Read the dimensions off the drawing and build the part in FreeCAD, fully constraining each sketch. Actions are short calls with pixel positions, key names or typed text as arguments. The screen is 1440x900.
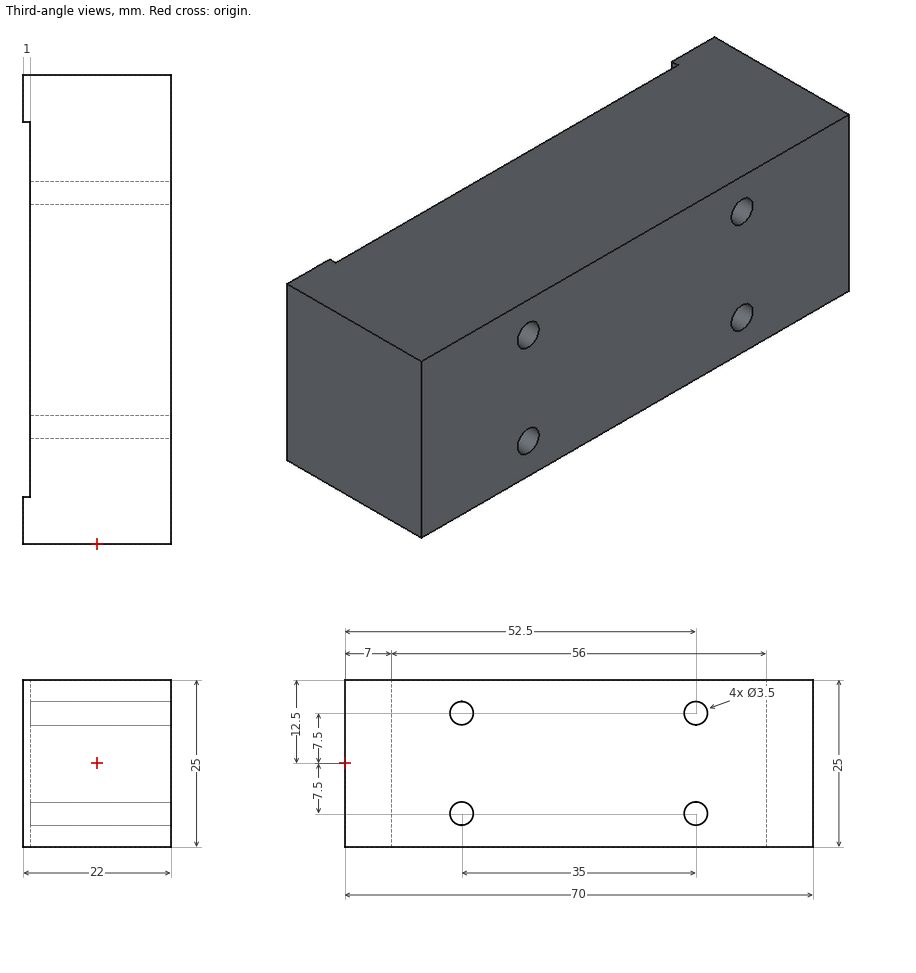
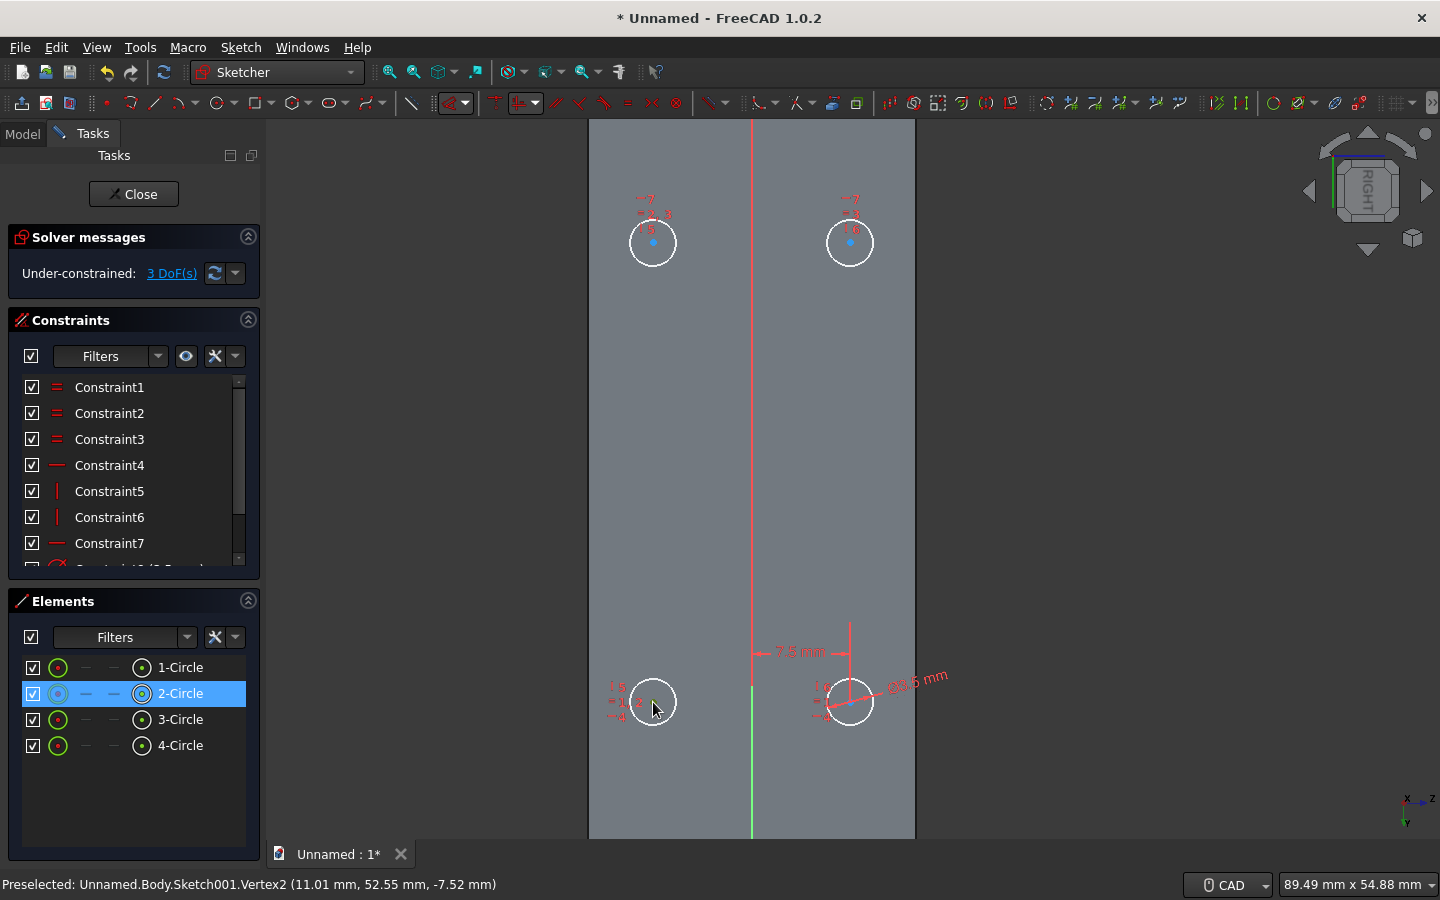
click(468, 104)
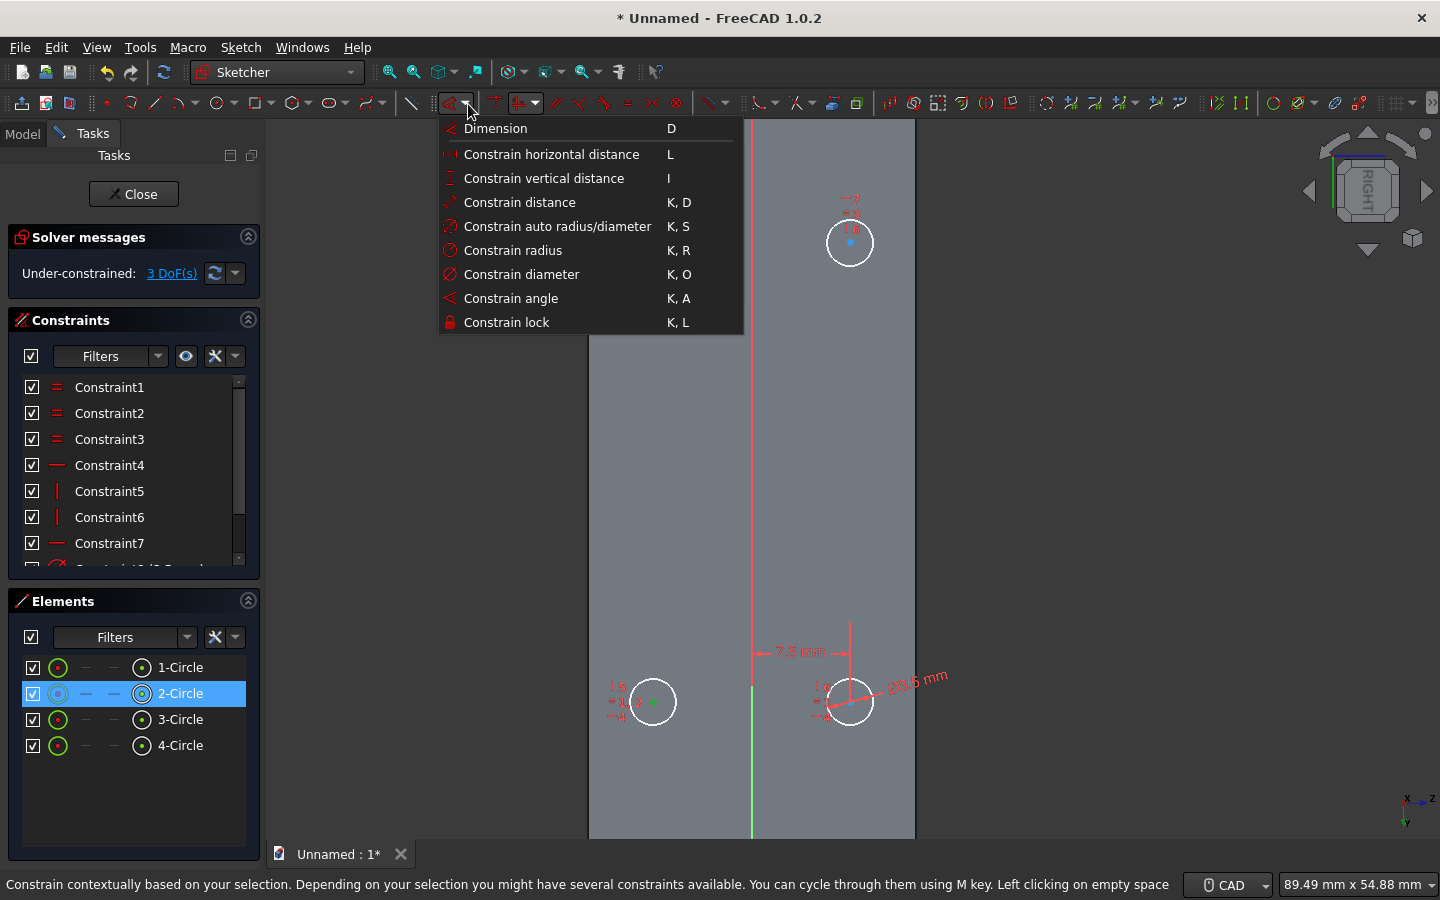
click(591, 154)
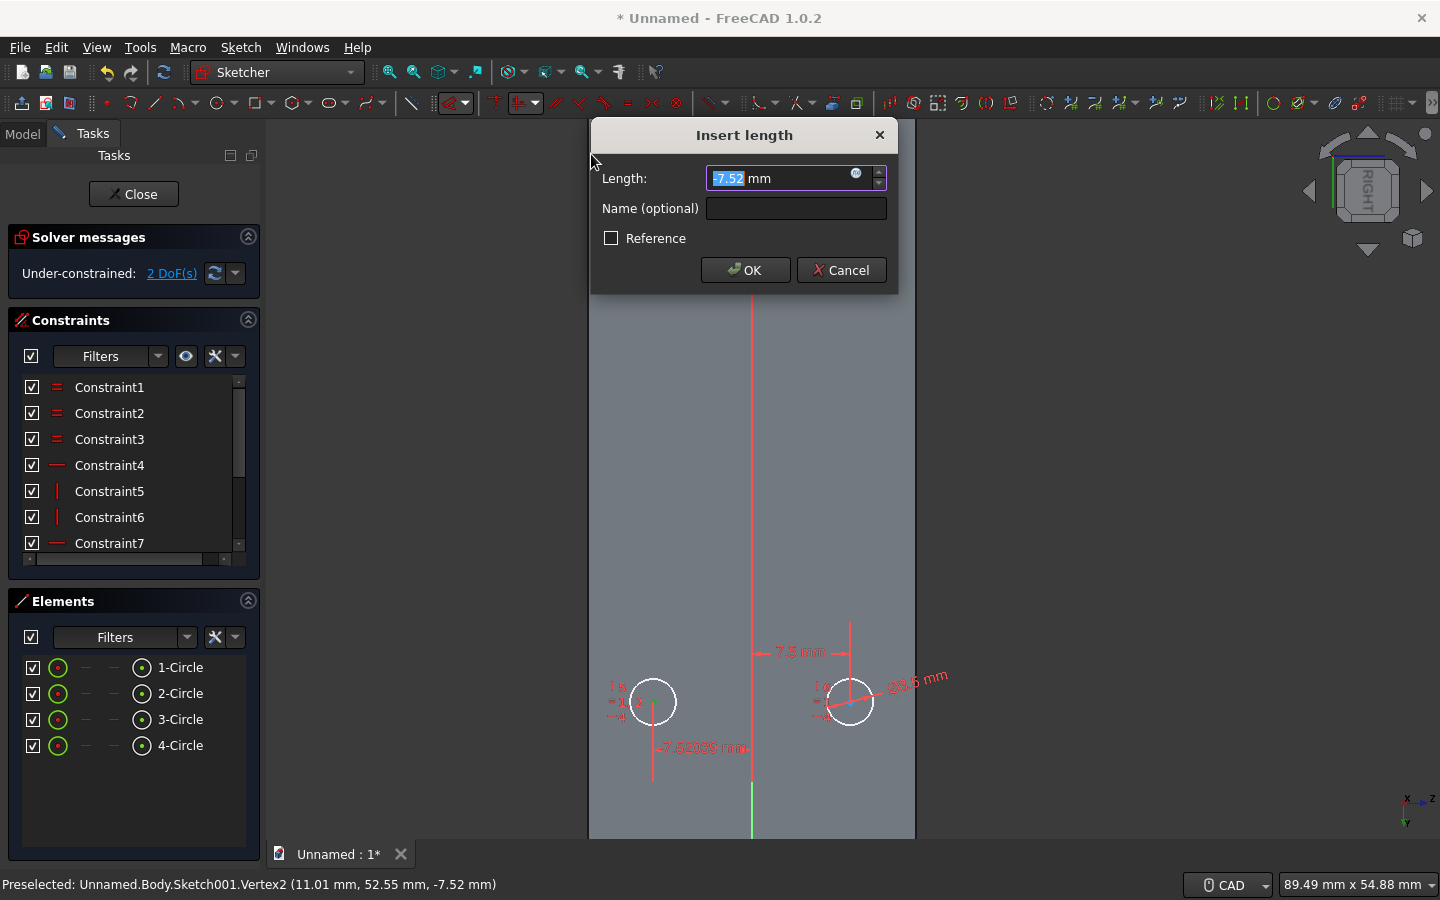
text(-7.5)
key(Return)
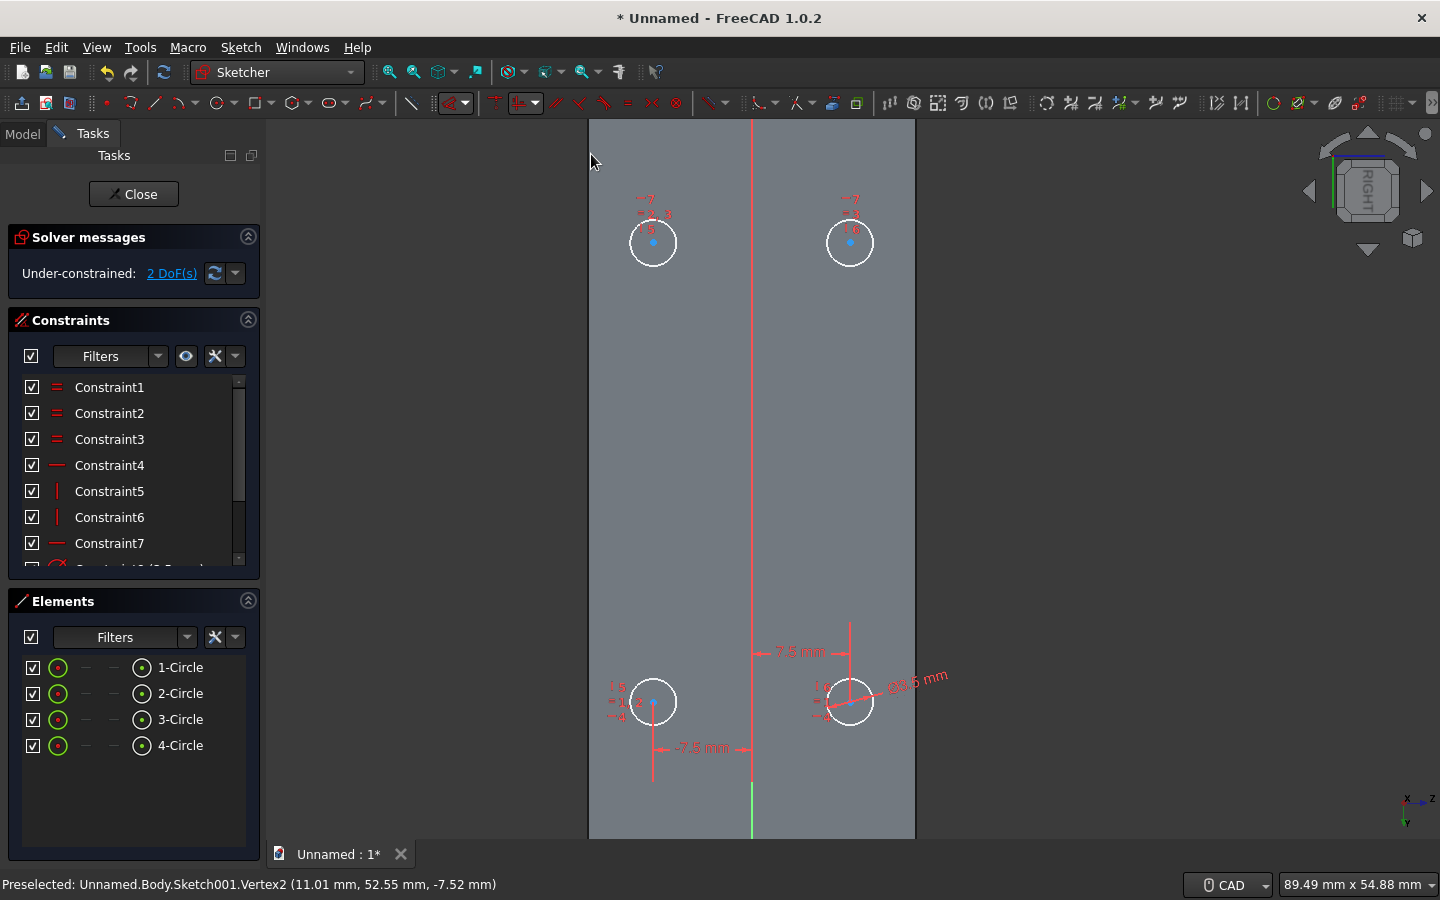
click(653, 702)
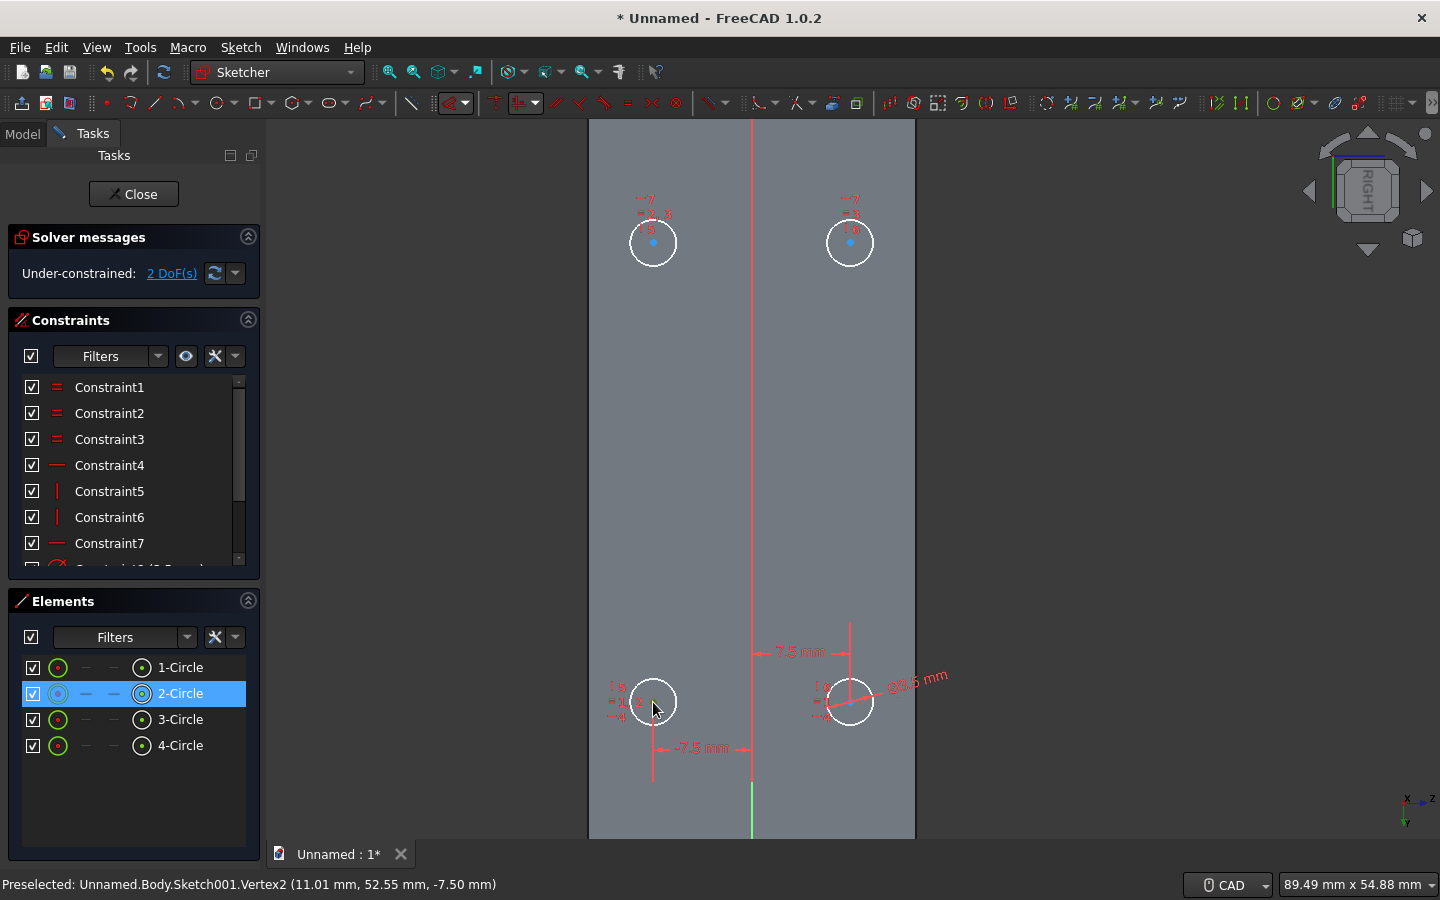
click(653, 243)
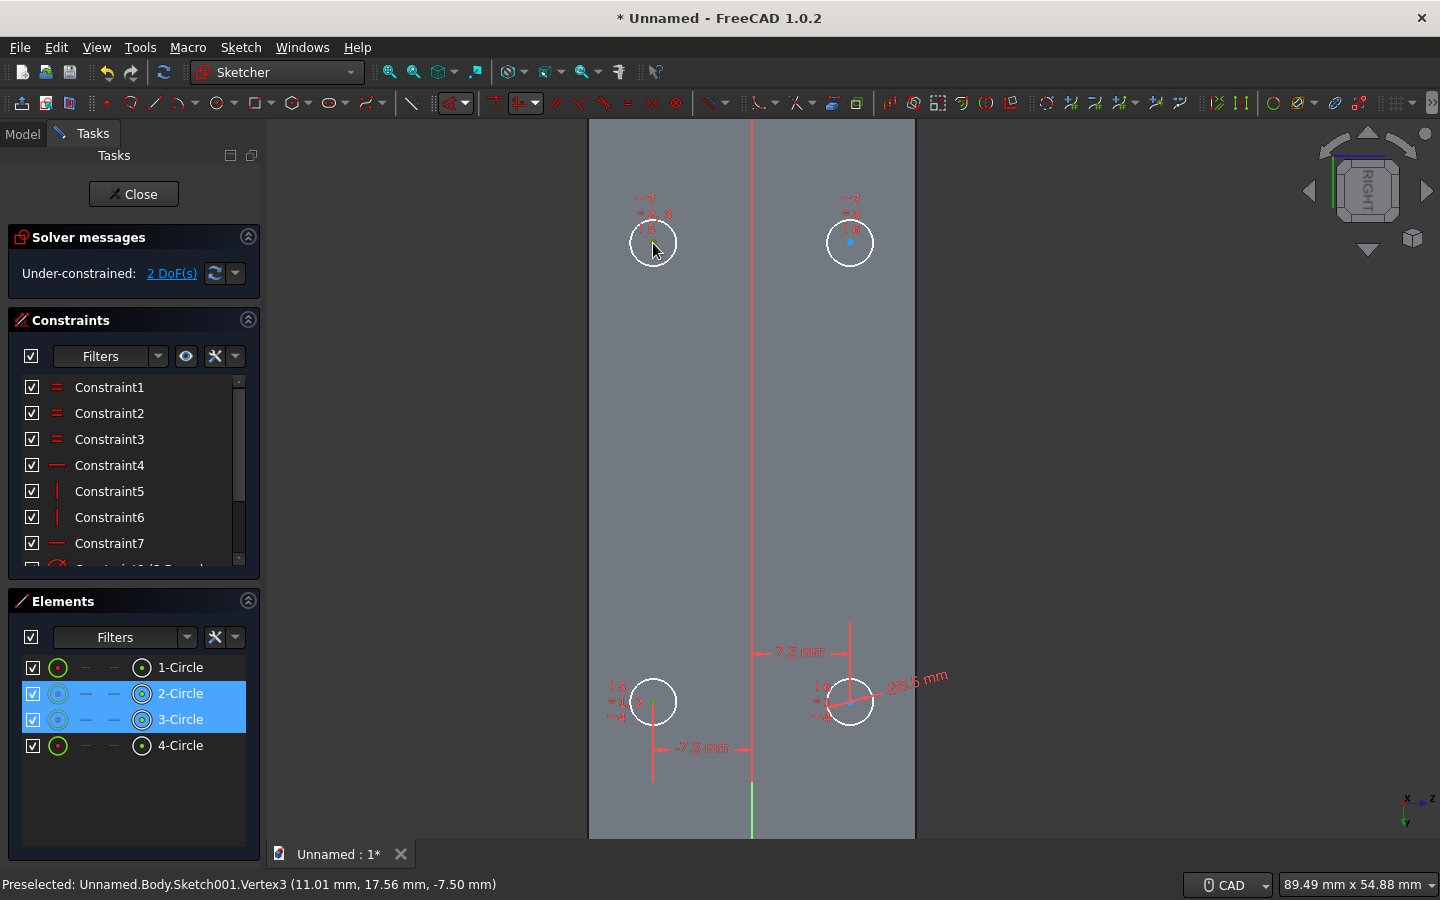
click(468, 104)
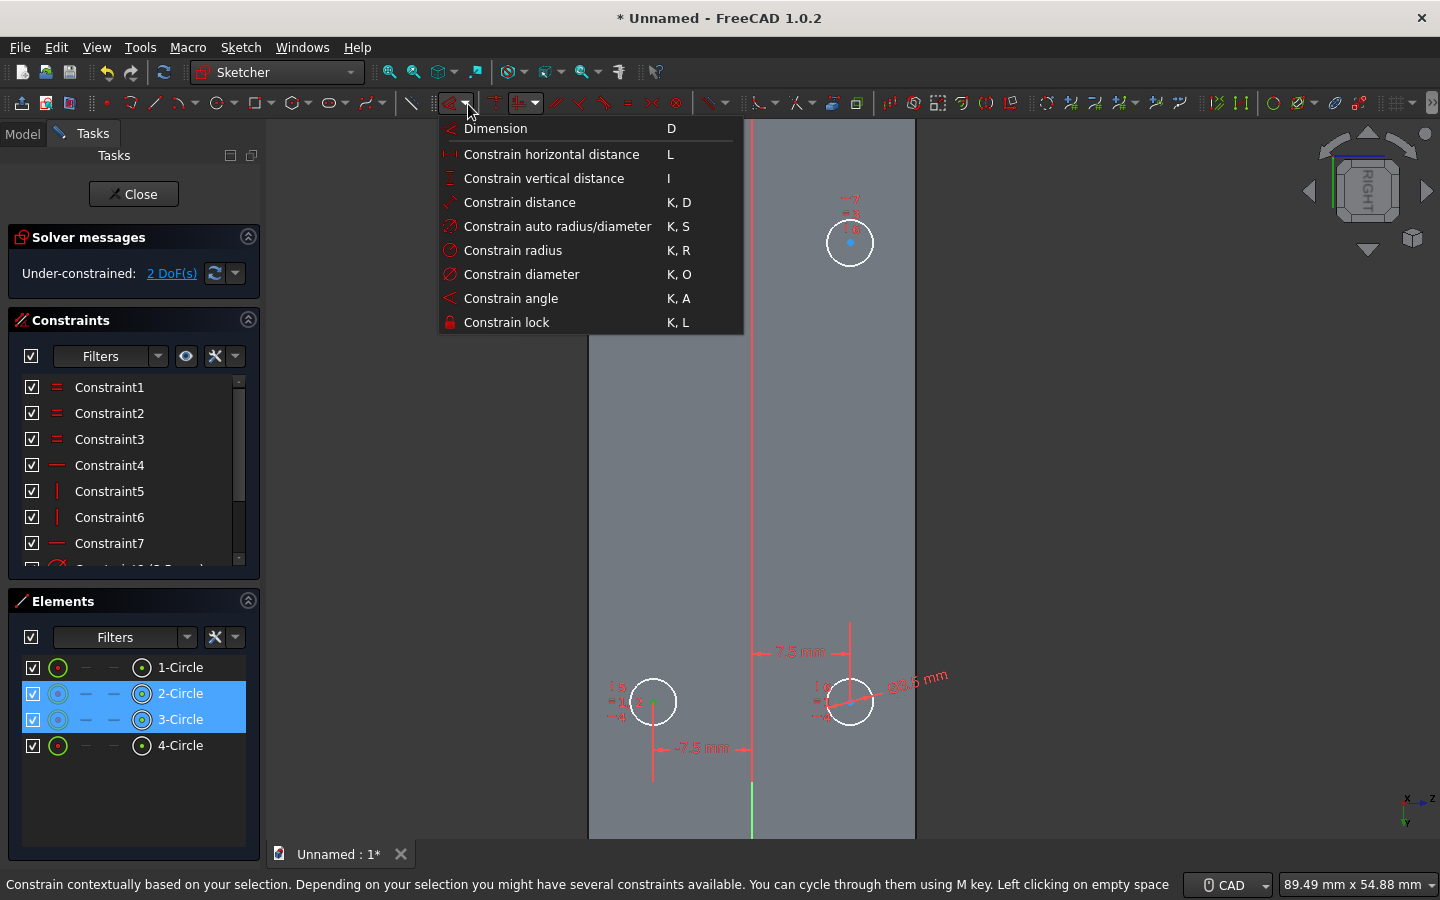
click(591, 178)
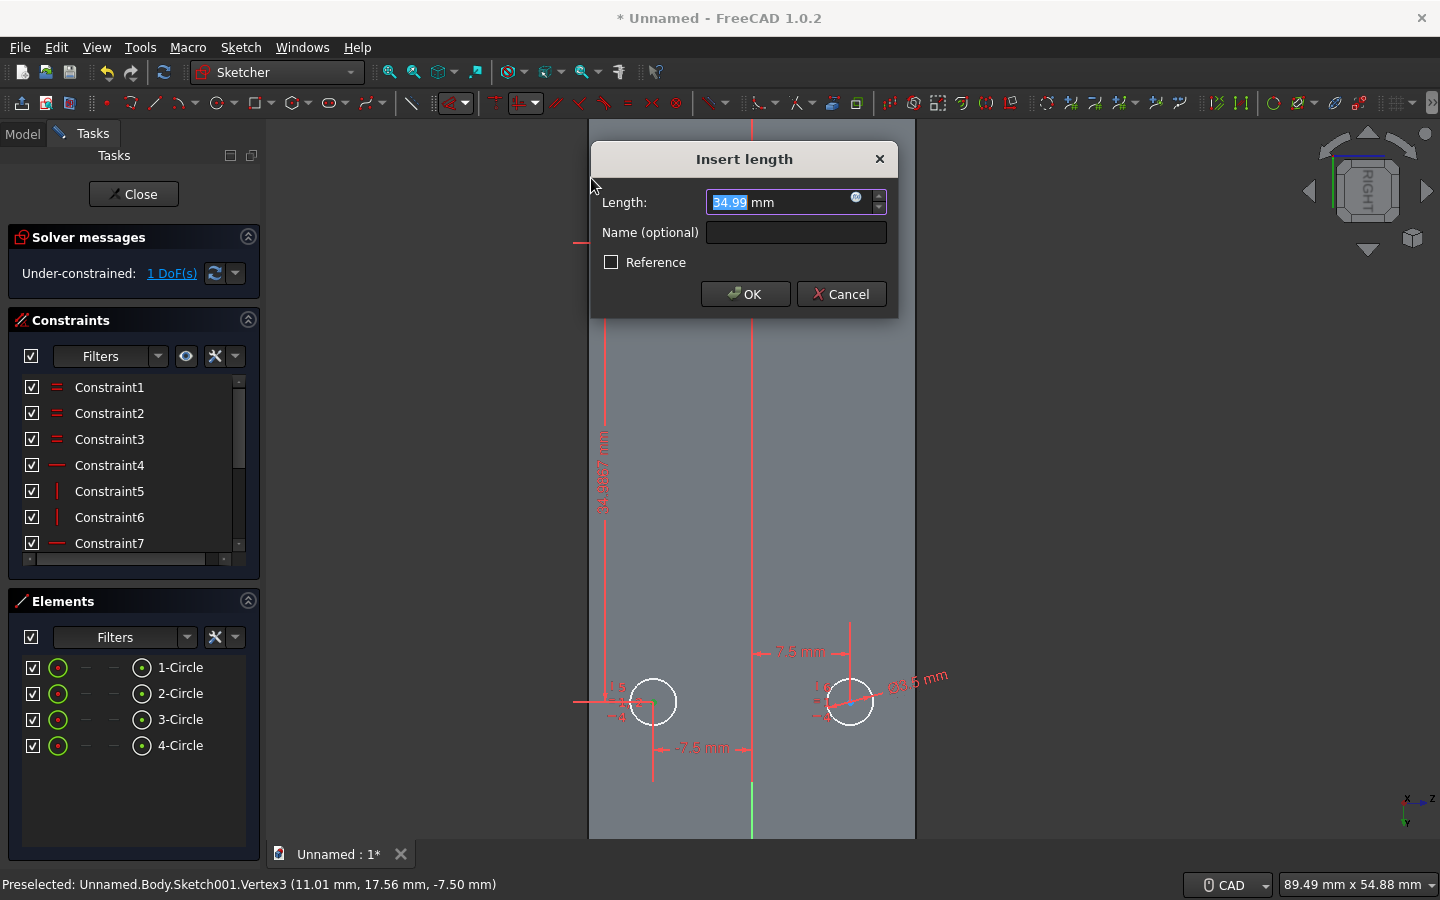
text(35)
key(Return)